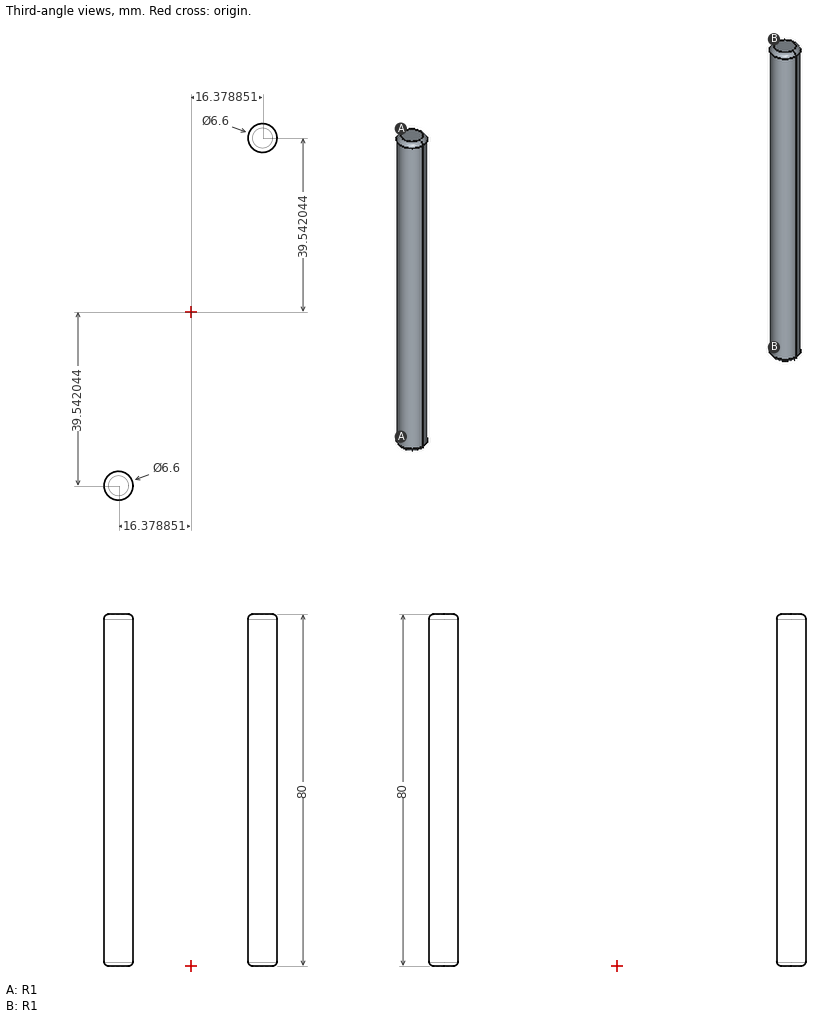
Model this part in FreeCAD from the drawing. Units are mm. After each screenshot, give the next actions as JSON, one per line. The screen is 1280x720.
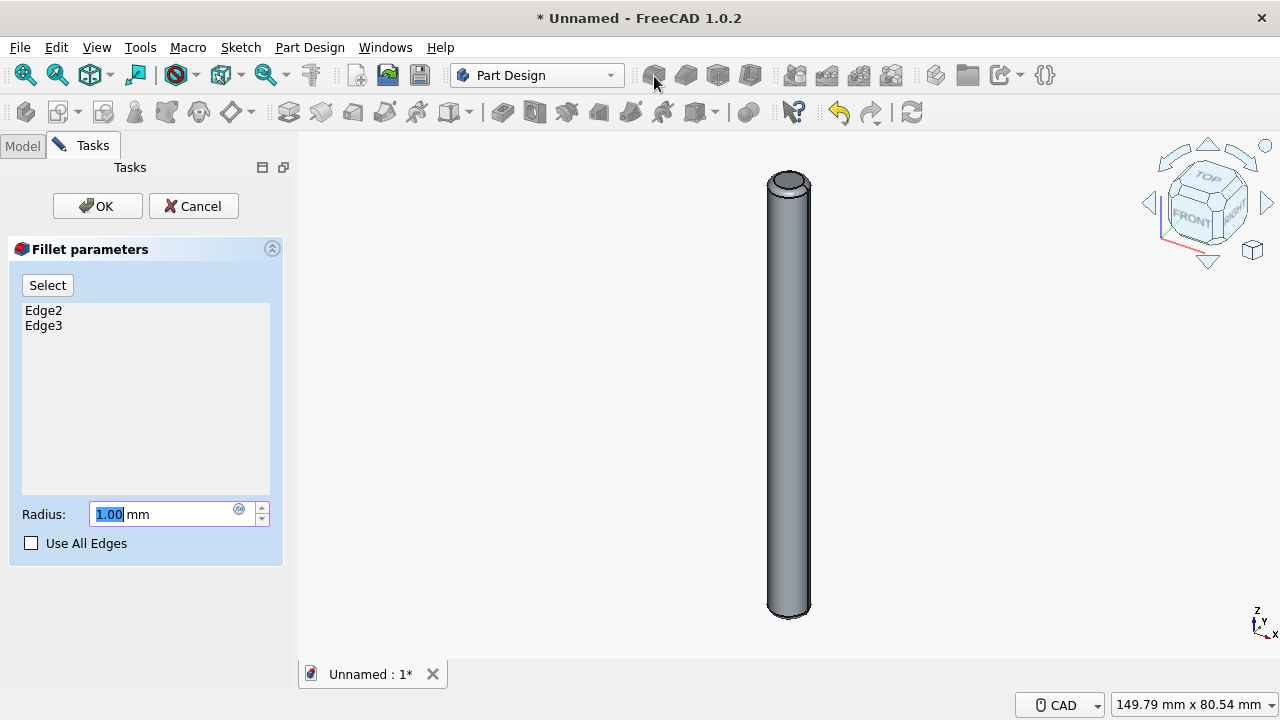
{"action": "type", "text": "1"}
{"action": "key", "text": "Tab"}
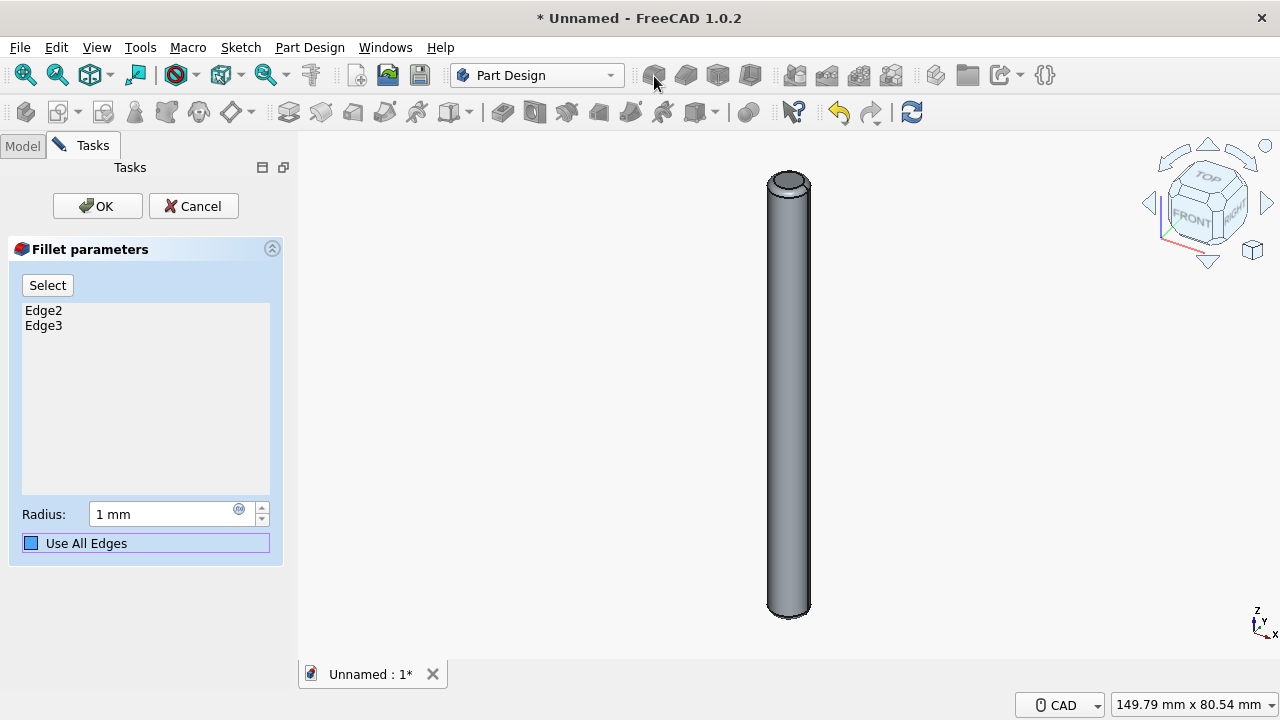
{"action": "left_click", "coordinate": [98, 206]}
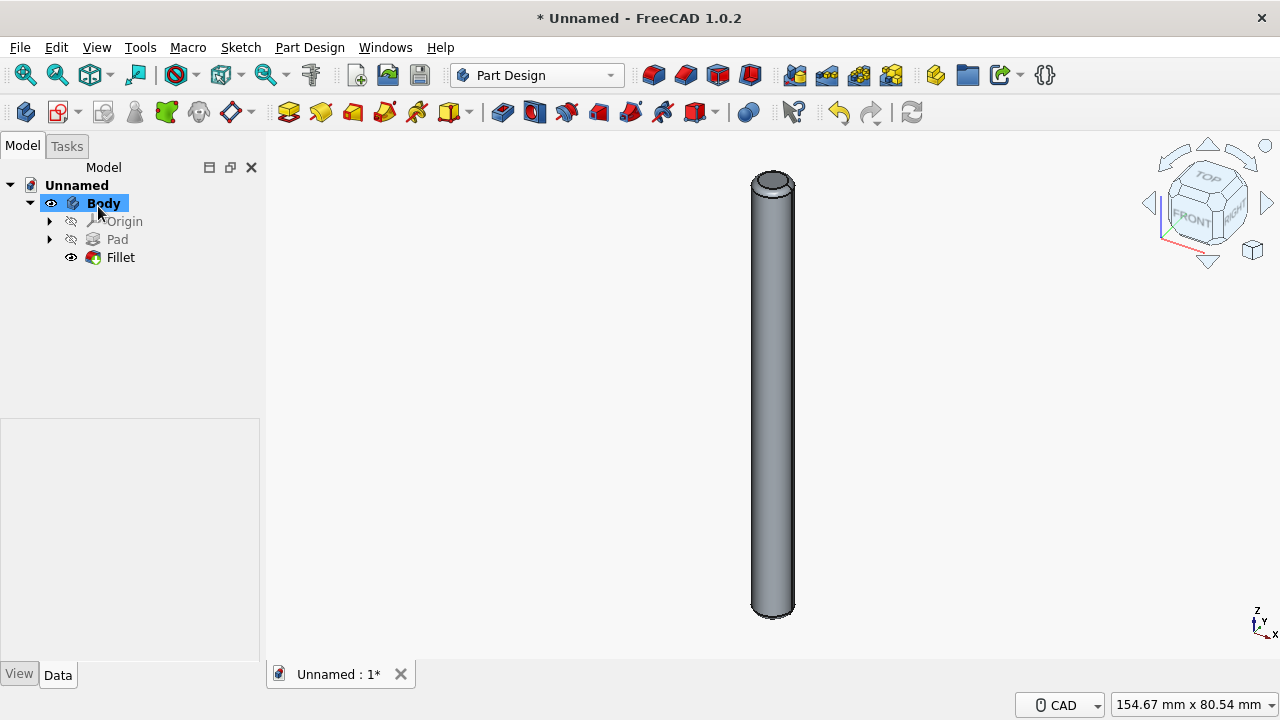
{"action": "left_click", "coordinate": [26, 112]}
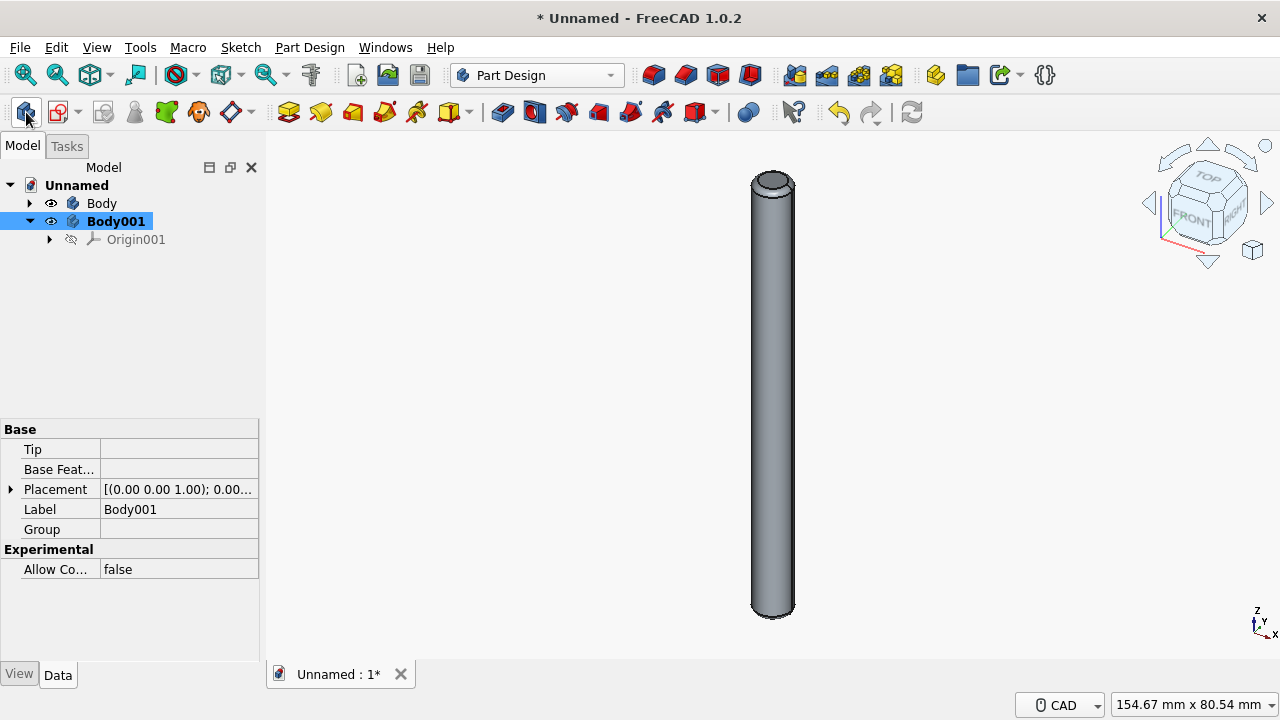
{"action": "left_click", "coordinate": [306, 619]}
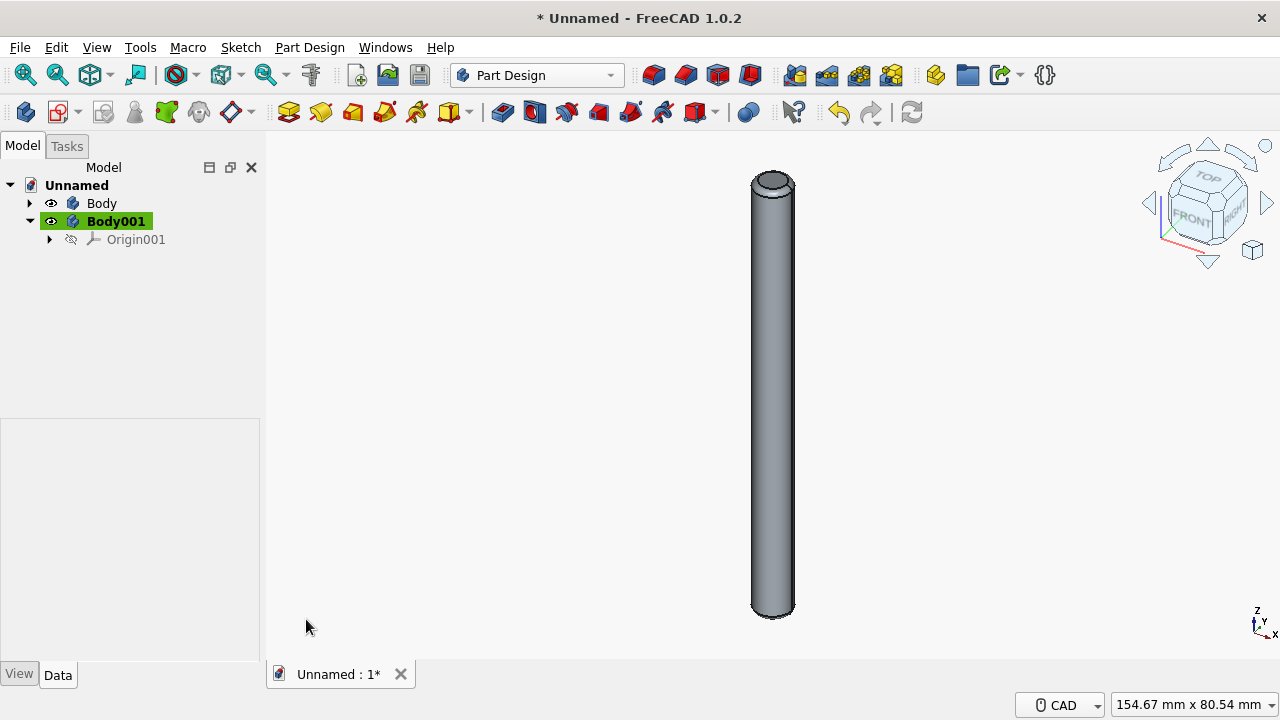
{"action": "left_click", "coordinate": [58, 112]}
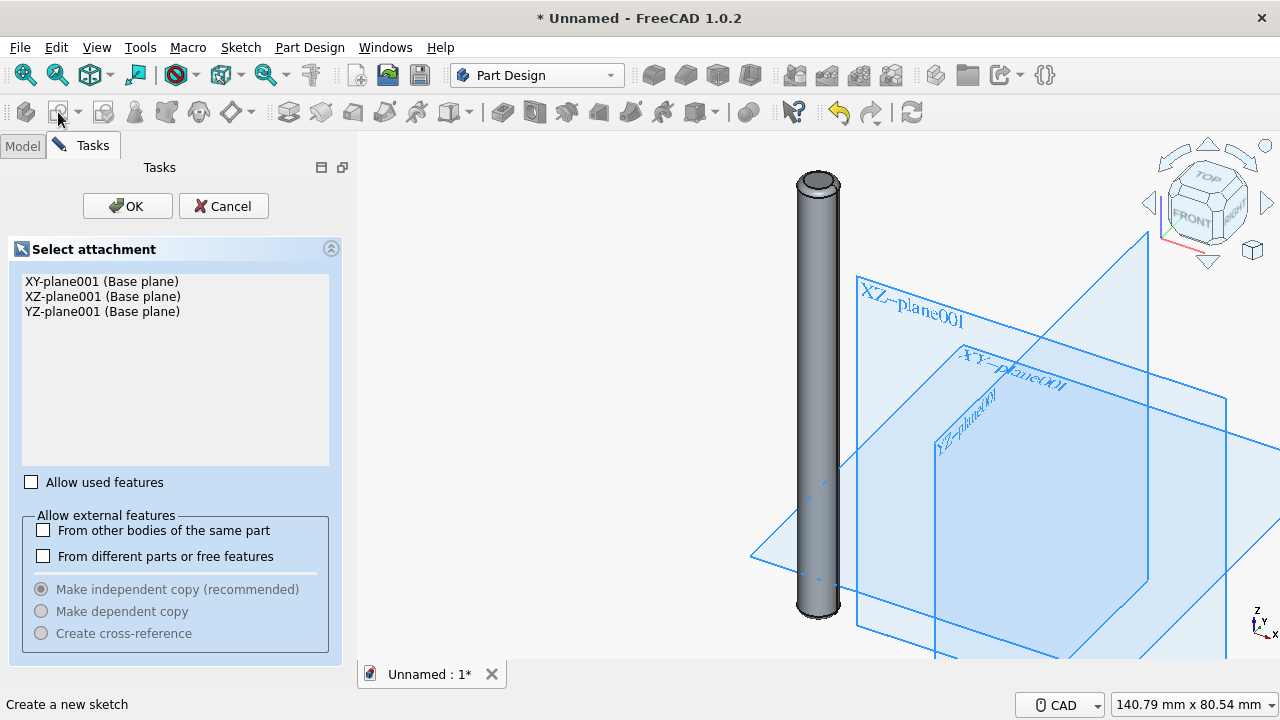
{"action": "left_click", "coordinate": [82, 282]}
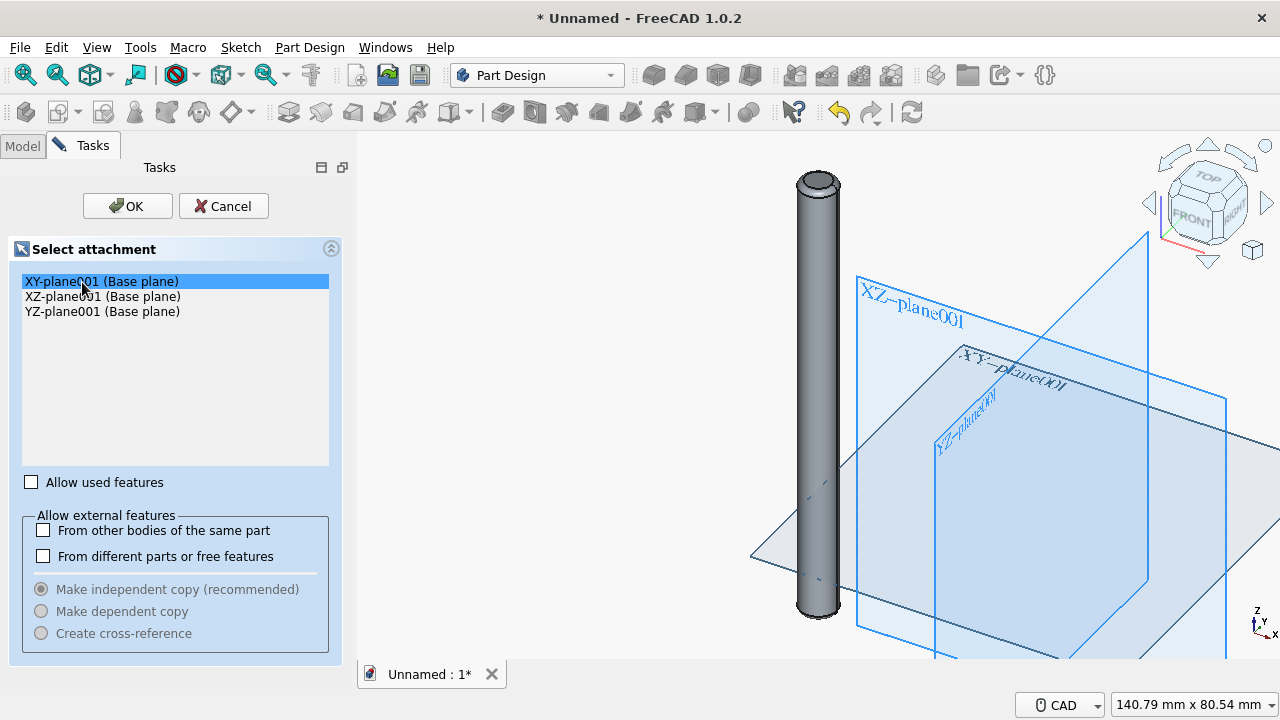
{"action": "left_click", "coordinate": [128, 206]}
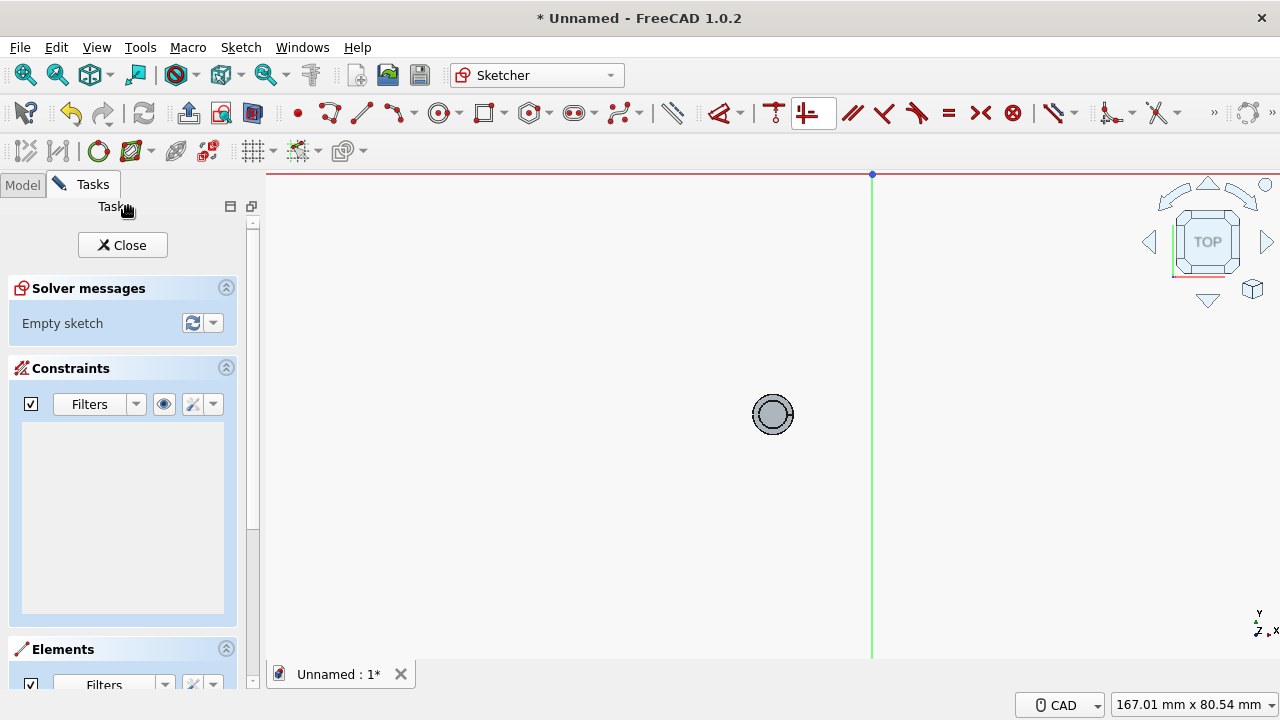
{"action": "scroll", "coordinate": [704, 414], "scroll_direction": "down", "scroll_amount": 5}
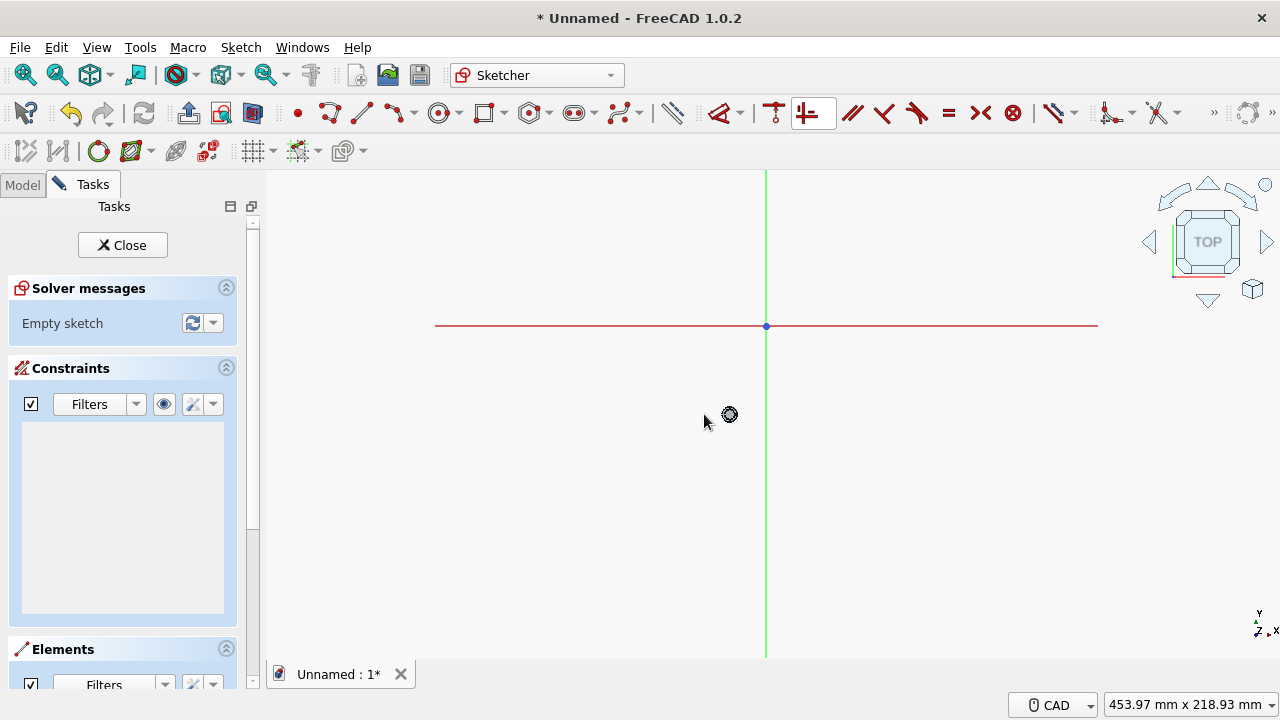
{"action": "scroll", "coordinate": [808, 229], "scroll_direction": "up", "scroll_amount": 15}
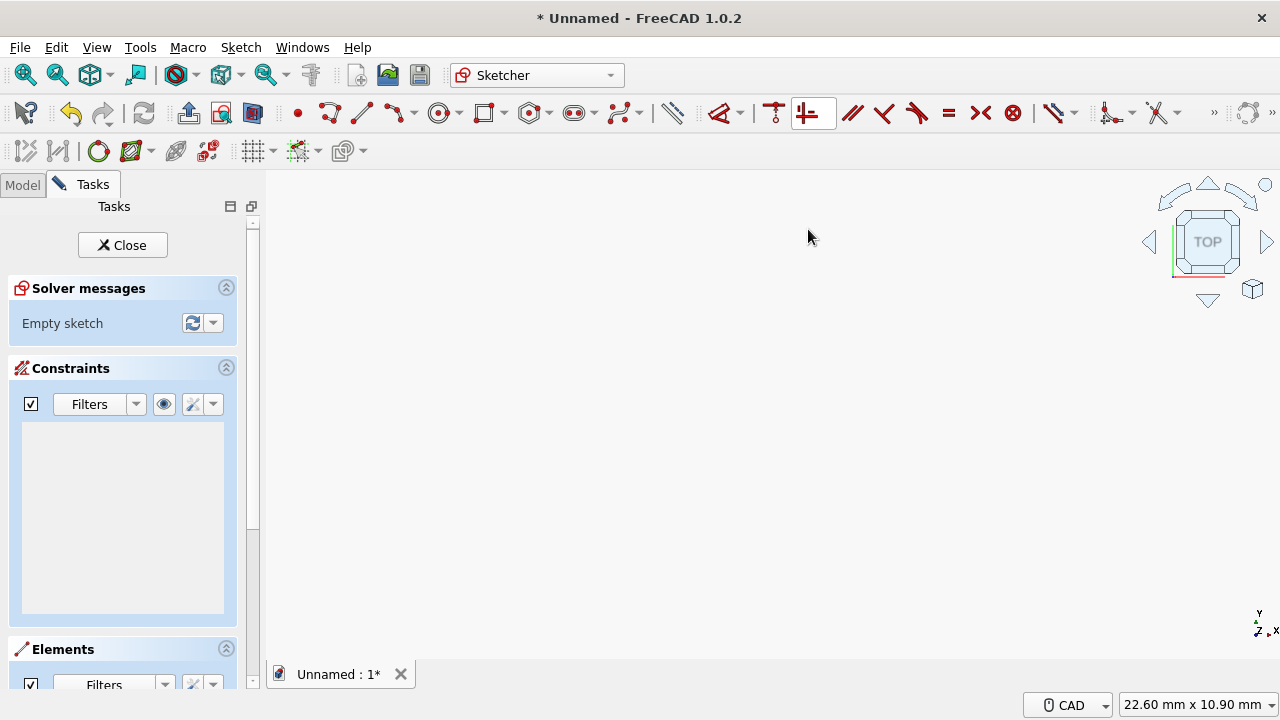
{"action": "key", "text": "g c"}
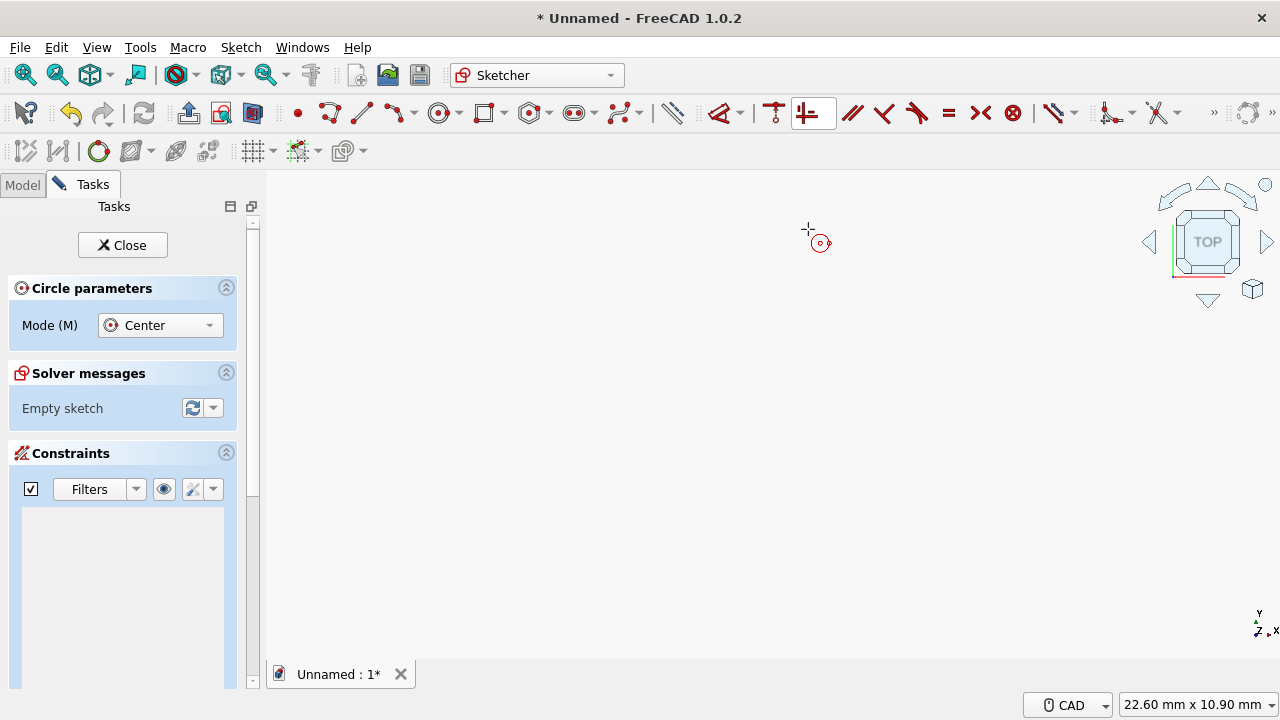
{"action": "left_click", "coordinate": [694, 405]}
{"action": "left_click", "coordinate": [799, 300]}
{"action": "key", "text": "Escape"}